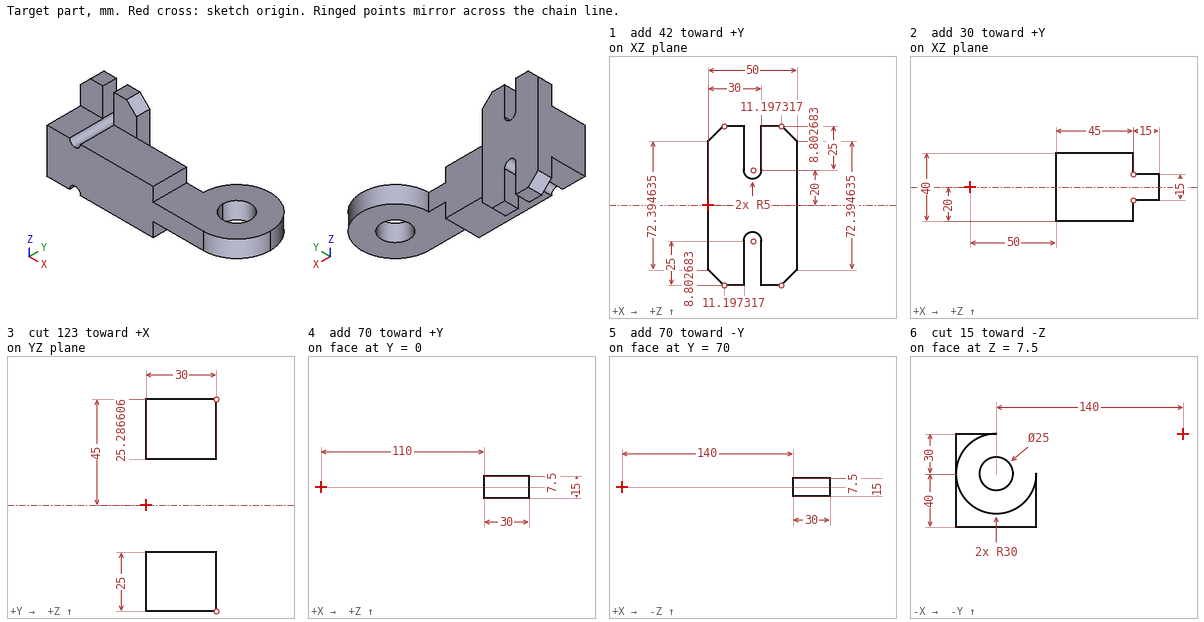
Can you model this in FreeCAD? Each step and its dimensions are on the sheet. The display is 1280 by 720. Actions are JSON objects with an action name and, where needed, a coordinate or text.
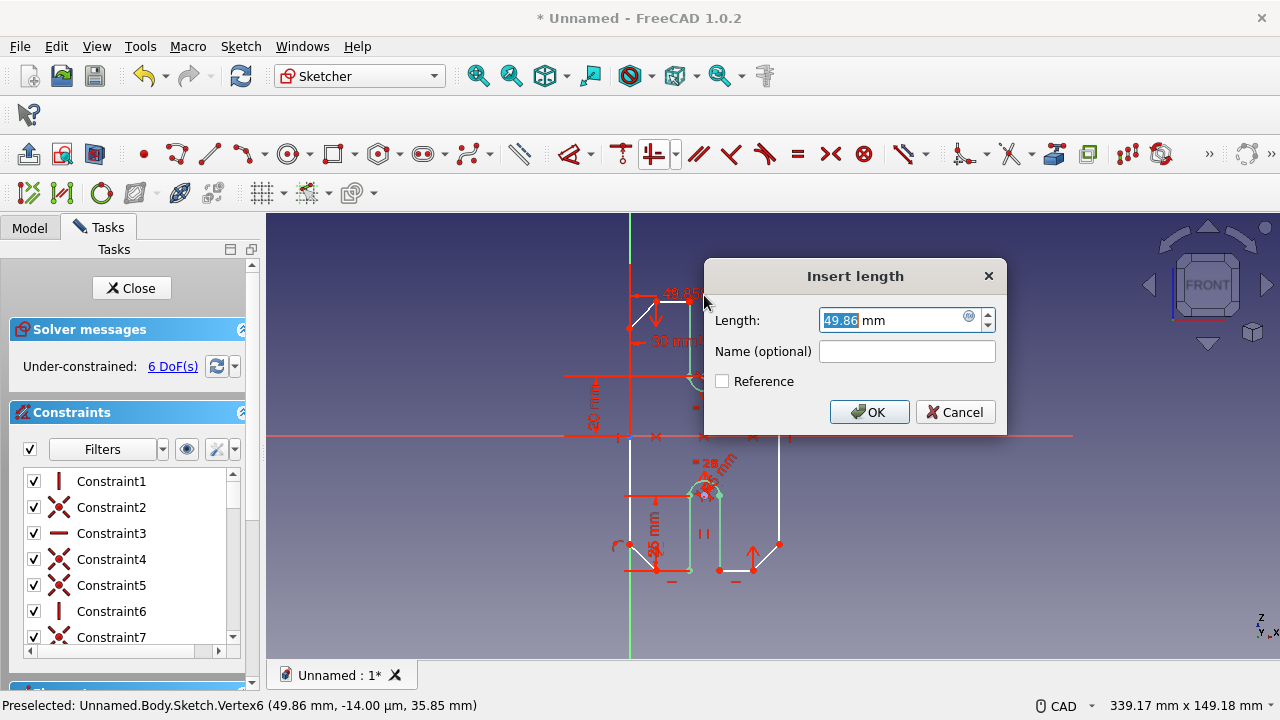
{"action": "type", "text": "50"}
{"action": "key", "text": "Return"}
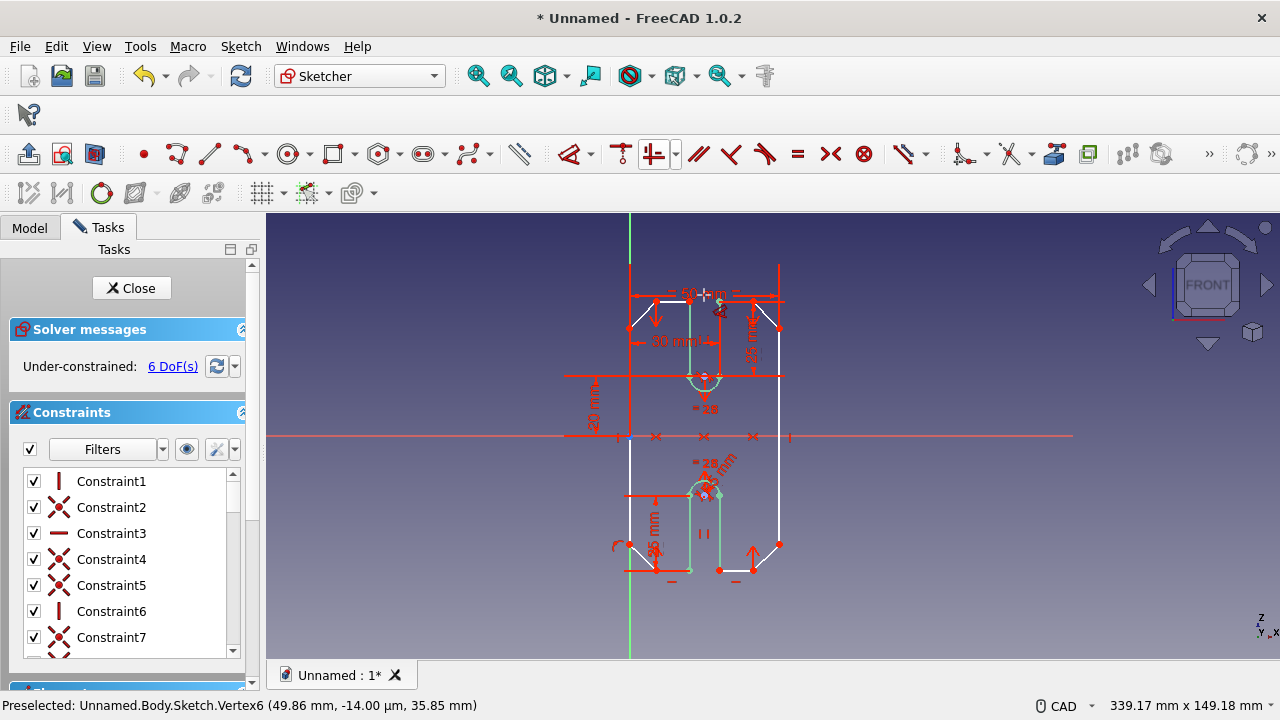
{"action": "scroll", "coordinate": [730, 302], "scroll_direction": "up", "scroll_amount": 2}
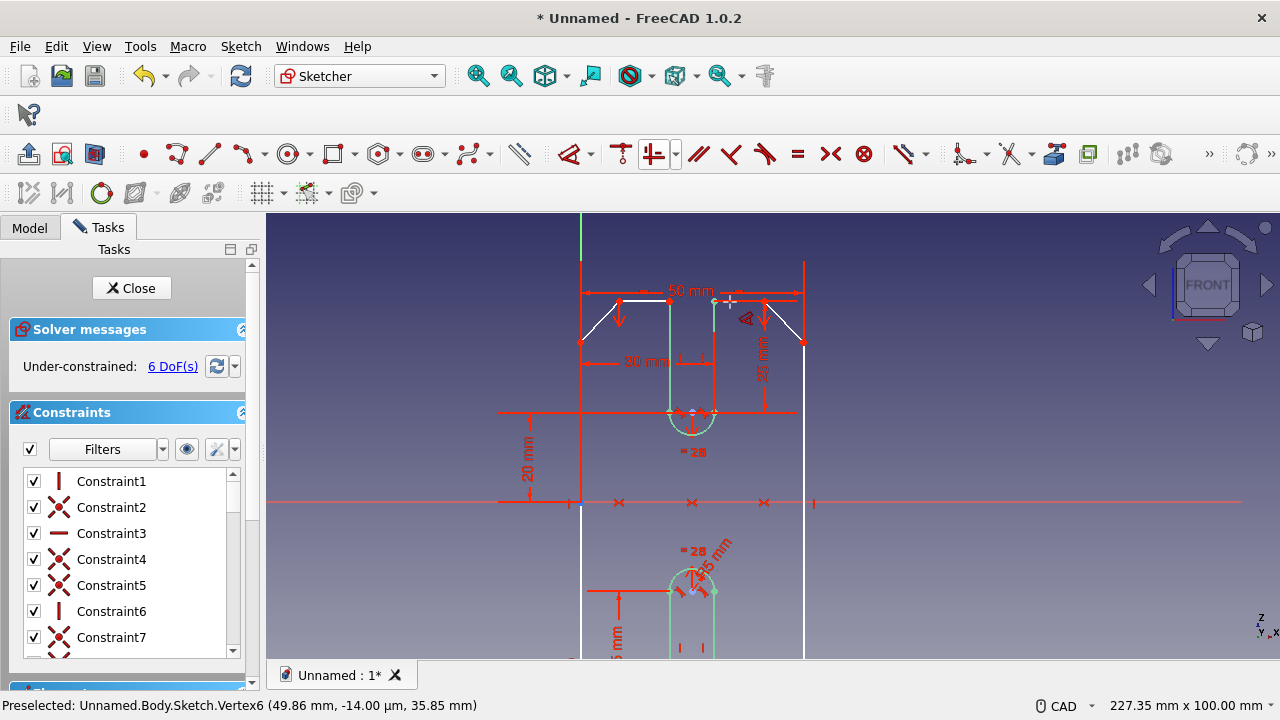
{"action": "left_click", "coordinate": [729, 301]}
{"action": "left_click", "coordinate": [739, 267]}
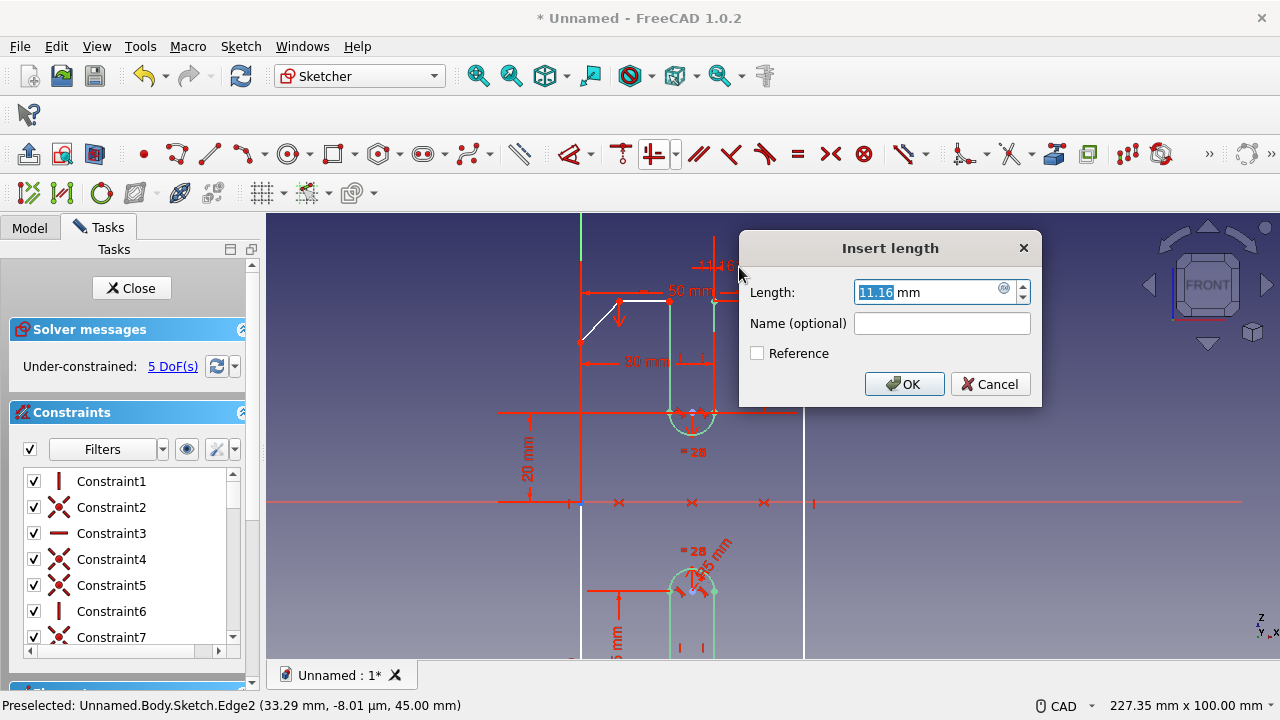
{"action": "type", "text": "11.197317"}
{"action": "key", "text": "Return"}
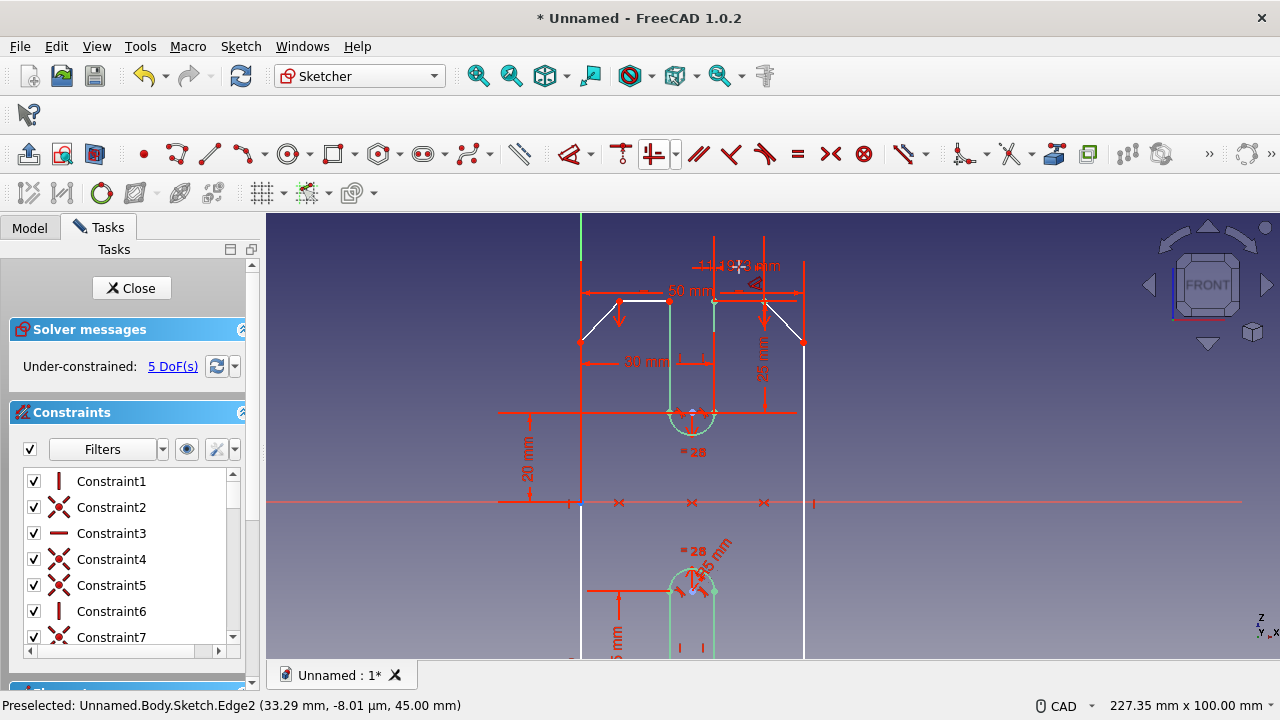
{"action": "left_click", "coordinate": [804, 439]}
{"action": "left_click", "coordinate": [838, 487]}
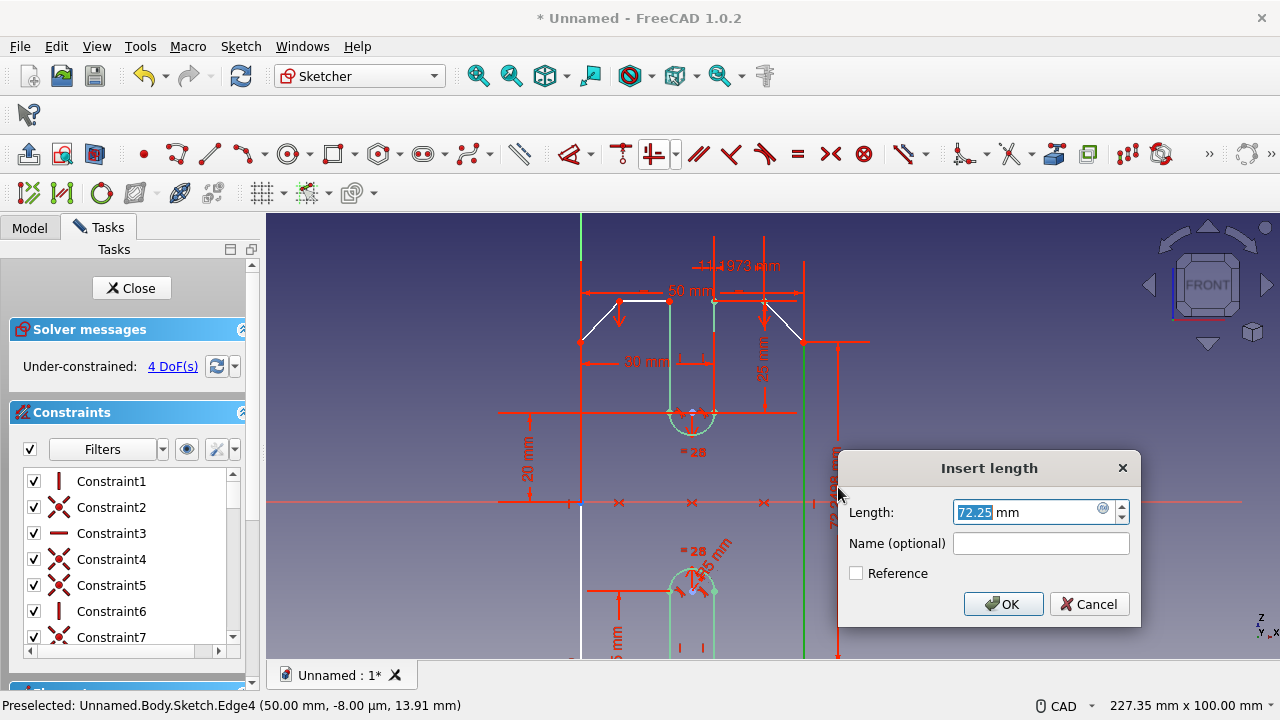
{"action": "type", "text": "72.394635"}
{"action": "key", "text": "Return"}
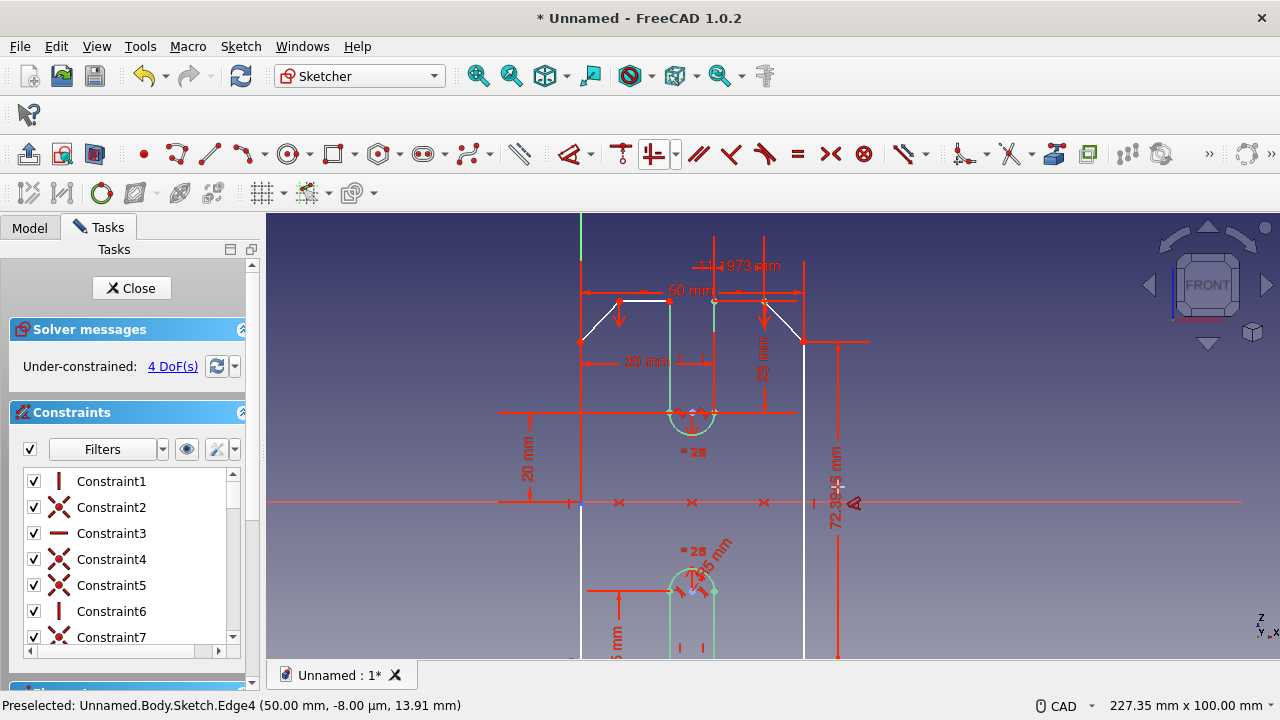
{"action": "scroll", "coordinate": [730, 302], "scroll_direction": "down", "scroll_amount": 2}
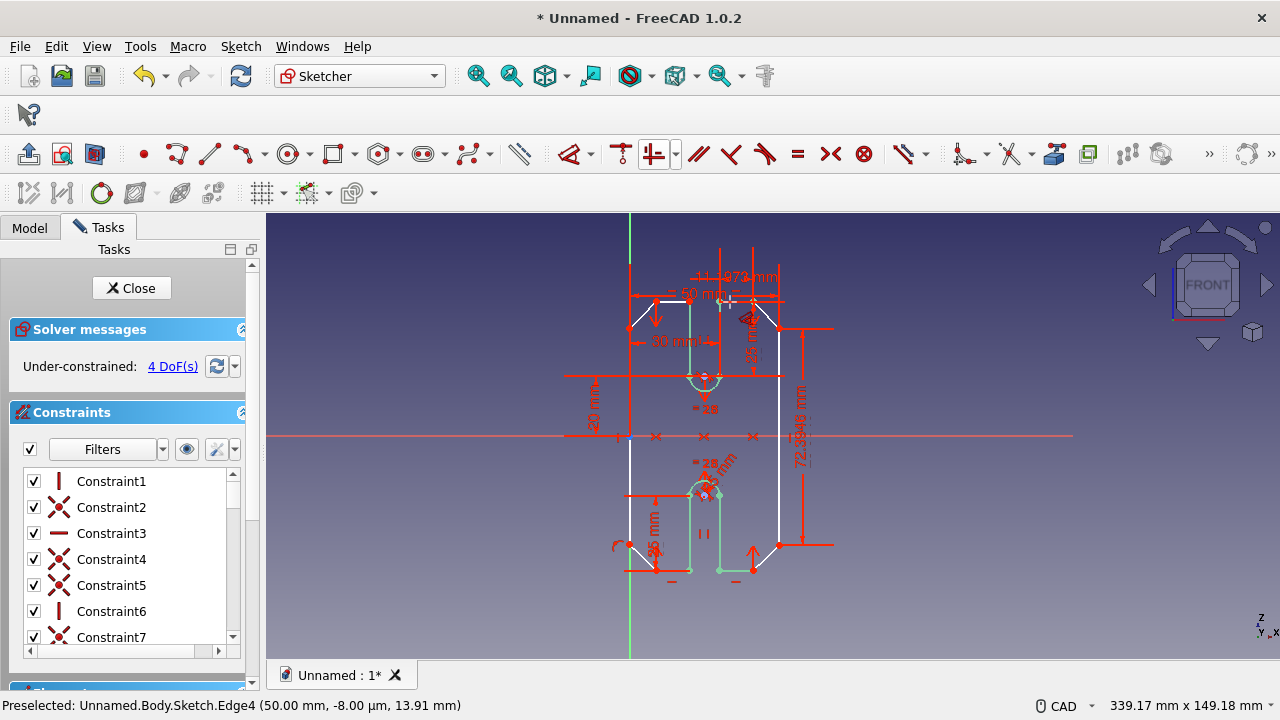
{"action": "scroll", "coordinate": [680, 571], "scroll_direction": "up", "scroll_amount": 2}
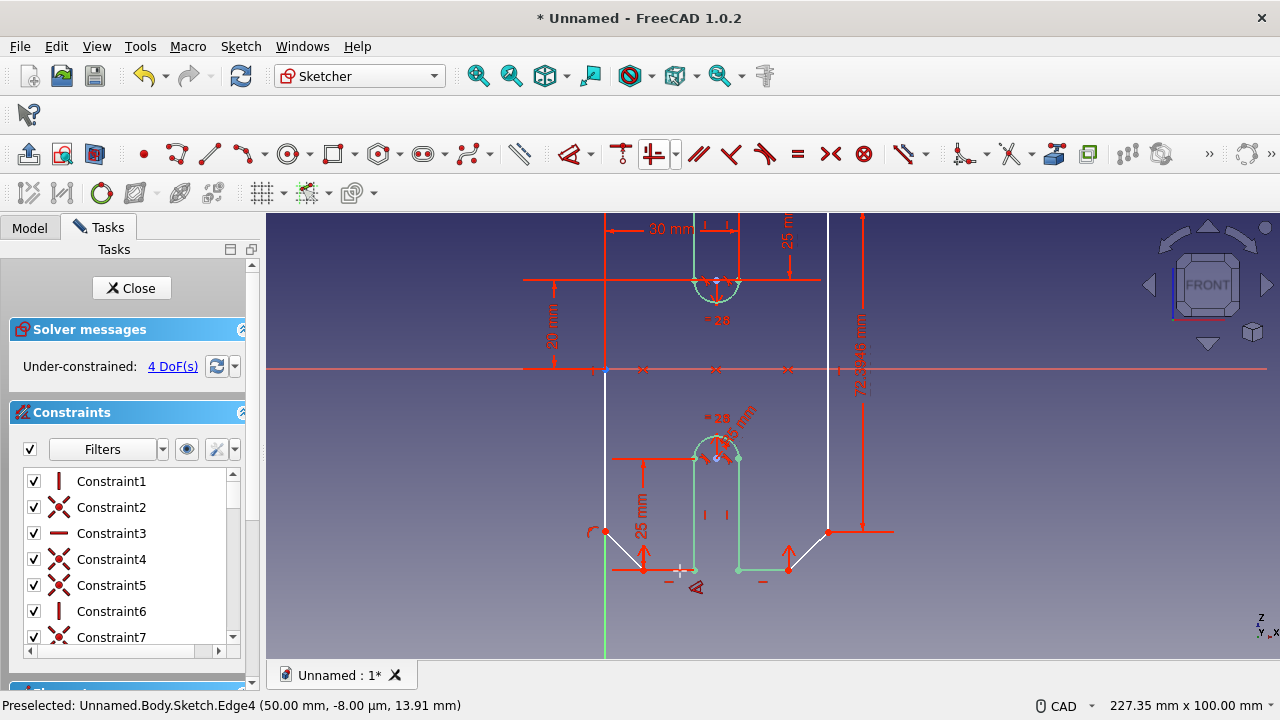
{"action": "left_click", "coordinate": [679, 570]}
{"action": "left_click", "coordinate": [669, 604]}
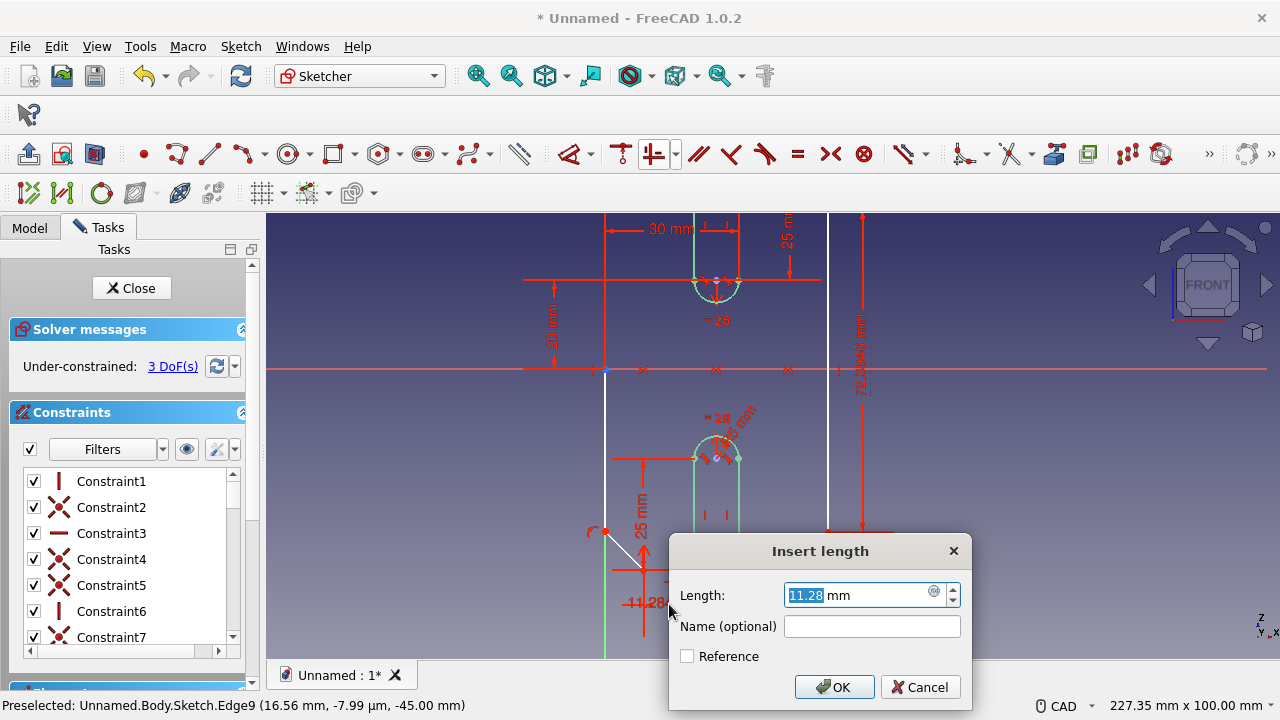
{"action": "type", "text": "11.197317"}
{"action": "key", "text": "Return"}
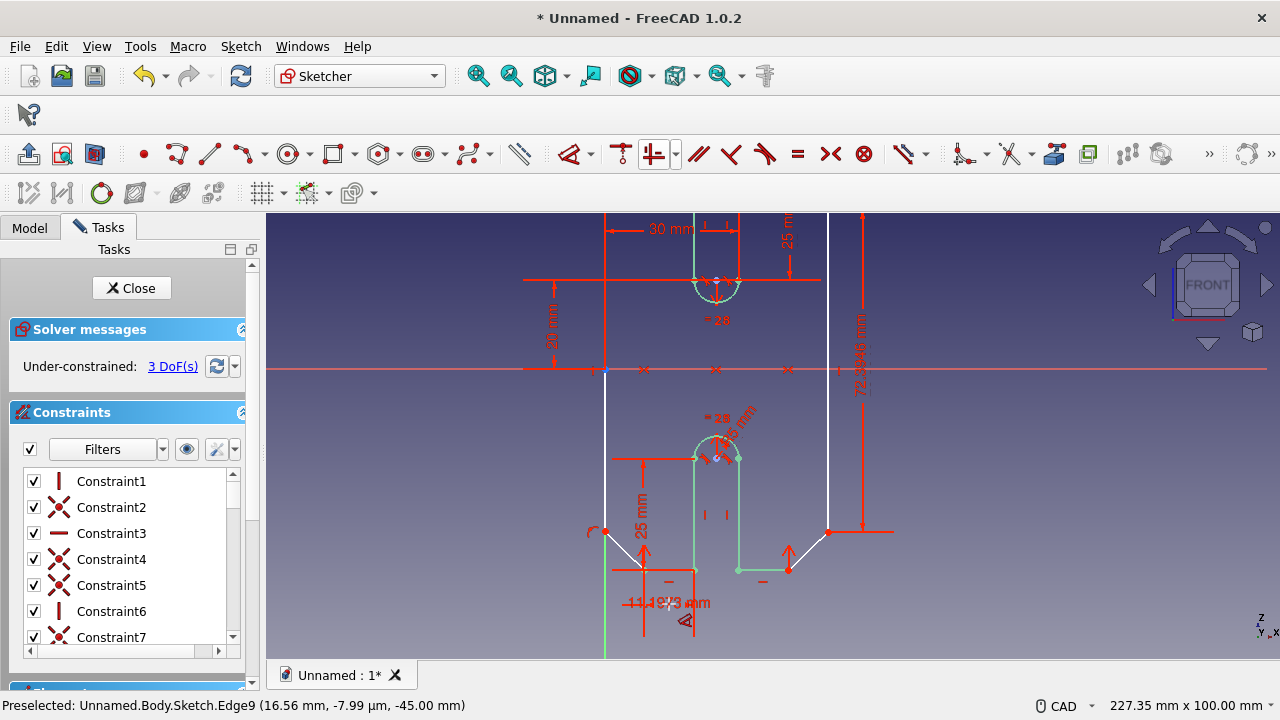
{"action": "left_click", "coordinate": [605, 435]}
{"action": "left_click", "coordinate": [571, 386]}